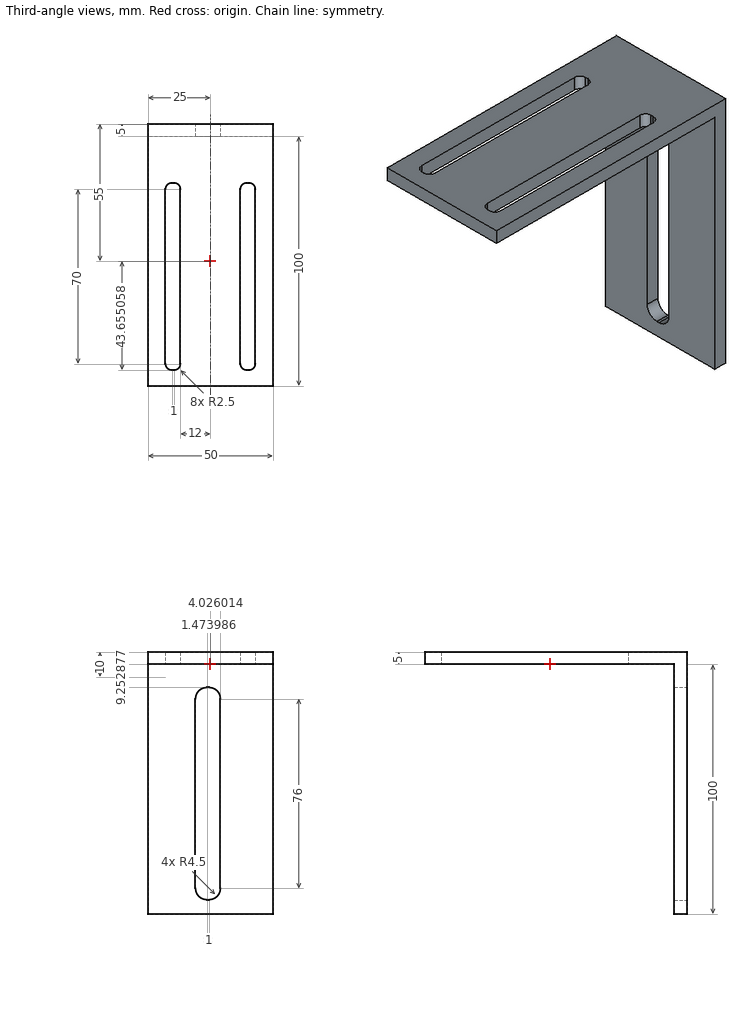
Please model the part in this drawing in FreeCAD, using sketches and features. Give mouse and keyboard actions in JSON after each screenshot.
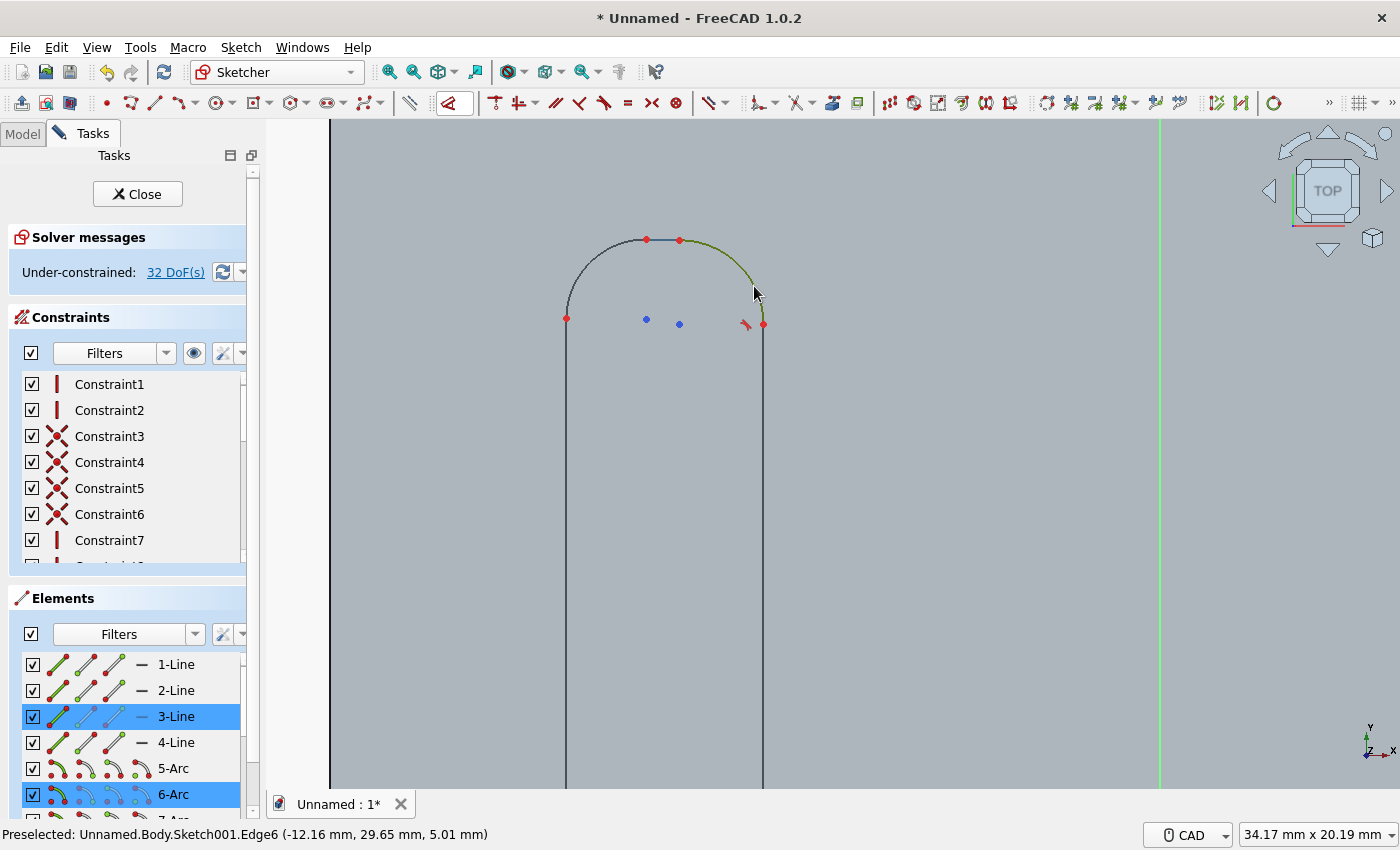
{"action": "key", "text": "t"}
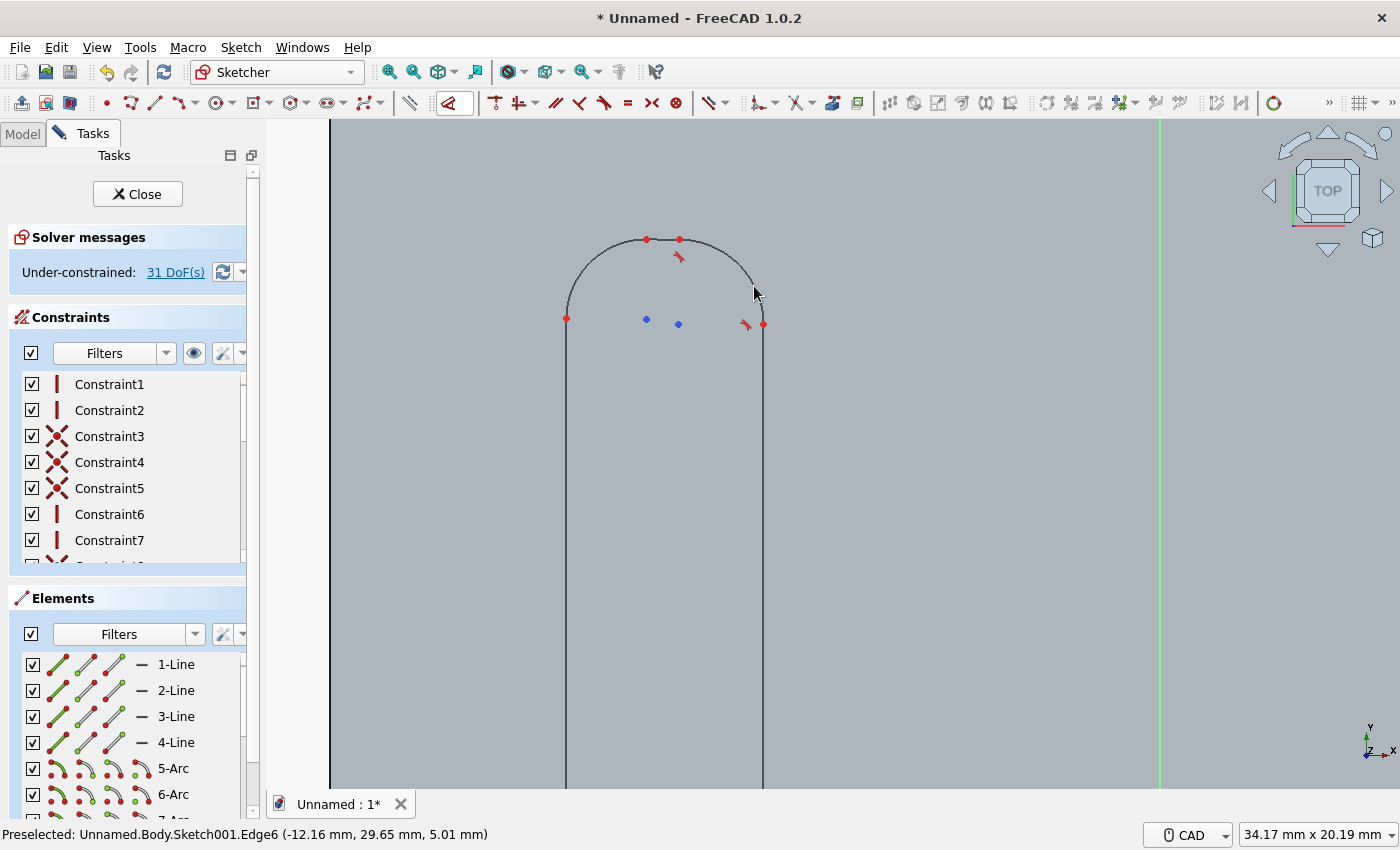
{"action": "scroll", "coordinate": [669, 240], "scroll_direction": "up", "scroll_amount": 2}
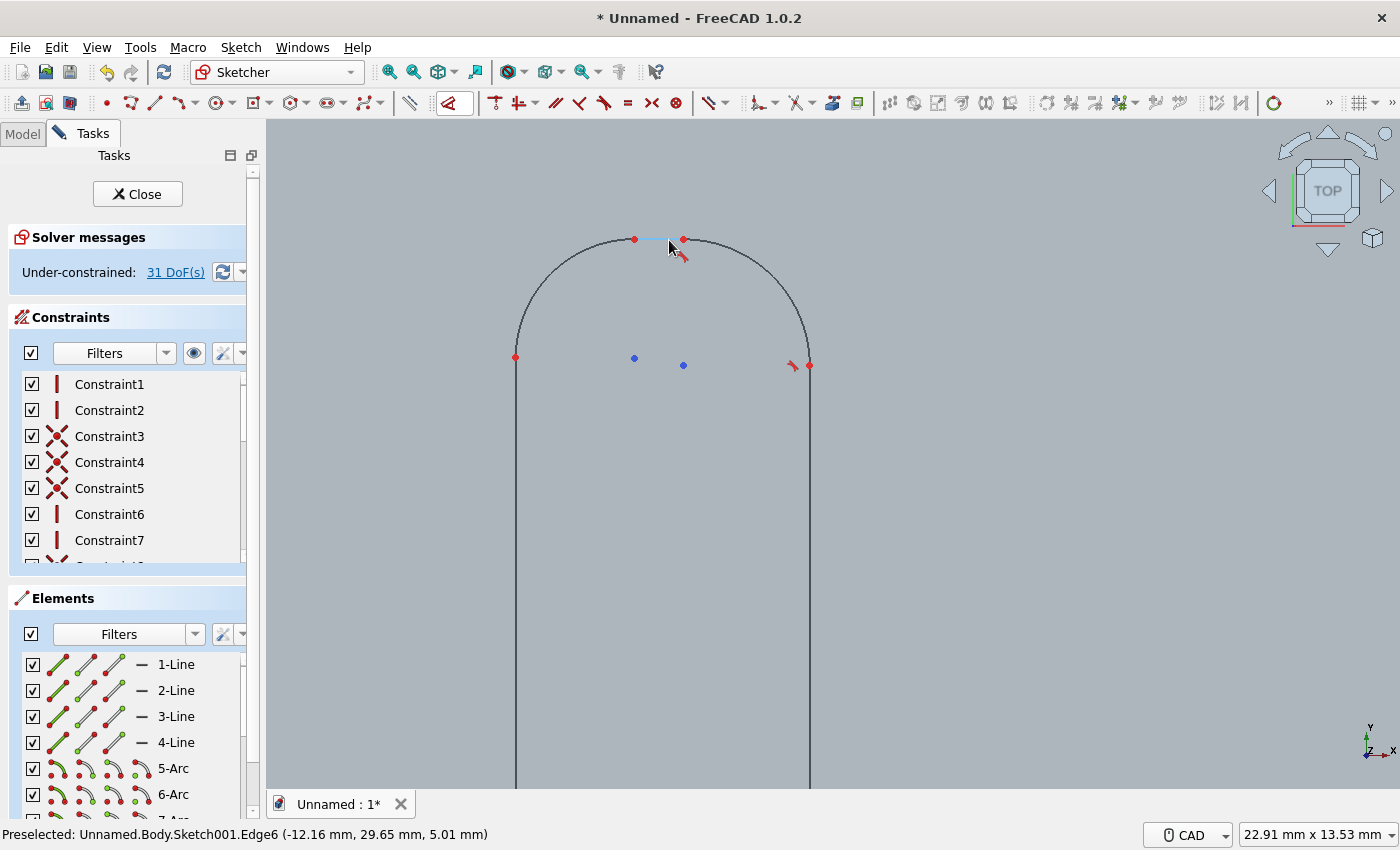
{"action": "left_click", "coordinate": [669, 239]}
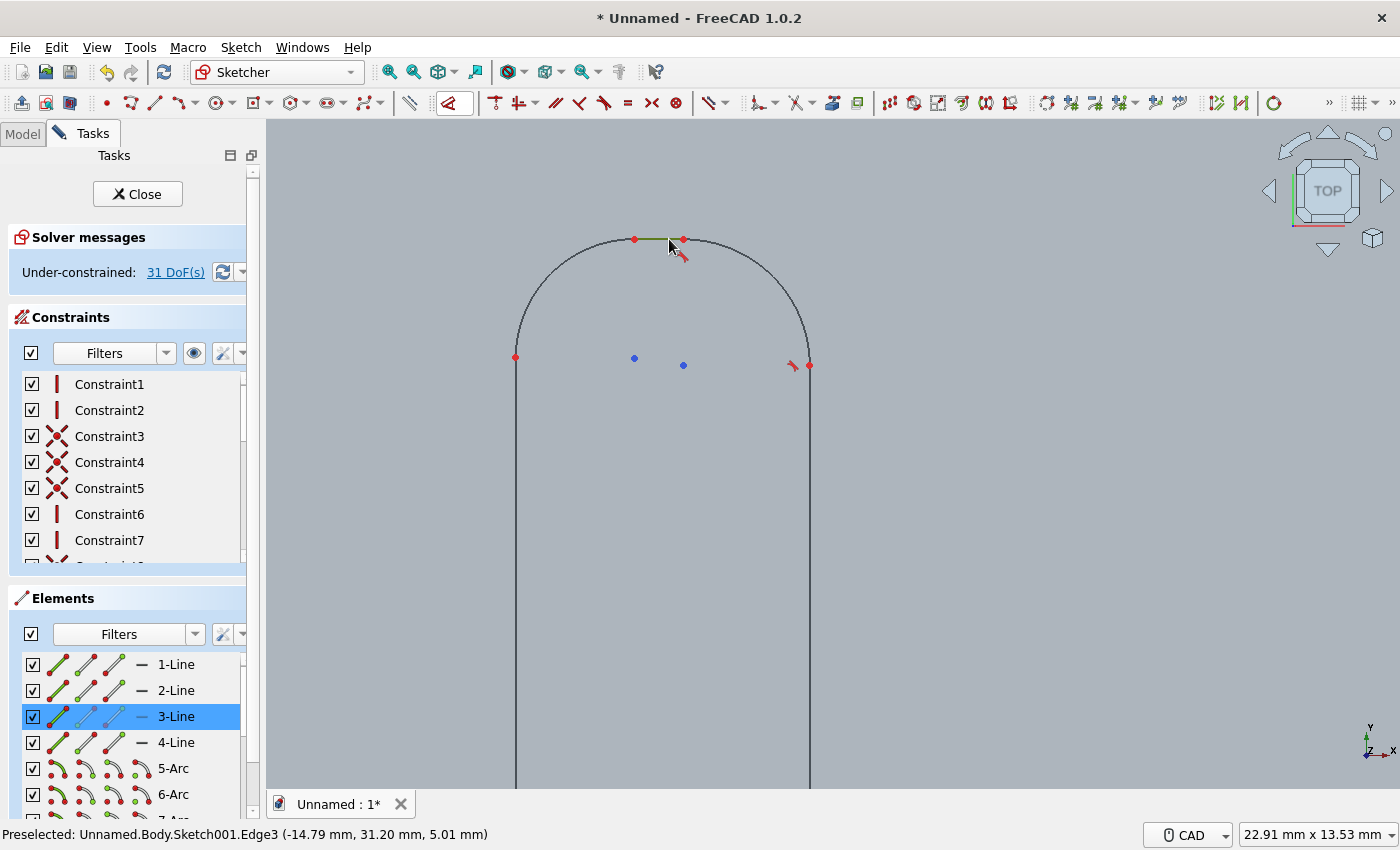
{"action": "scroll", "coordinate": [685, 250], "scroll_direction": "down", "scroll_amount": 11}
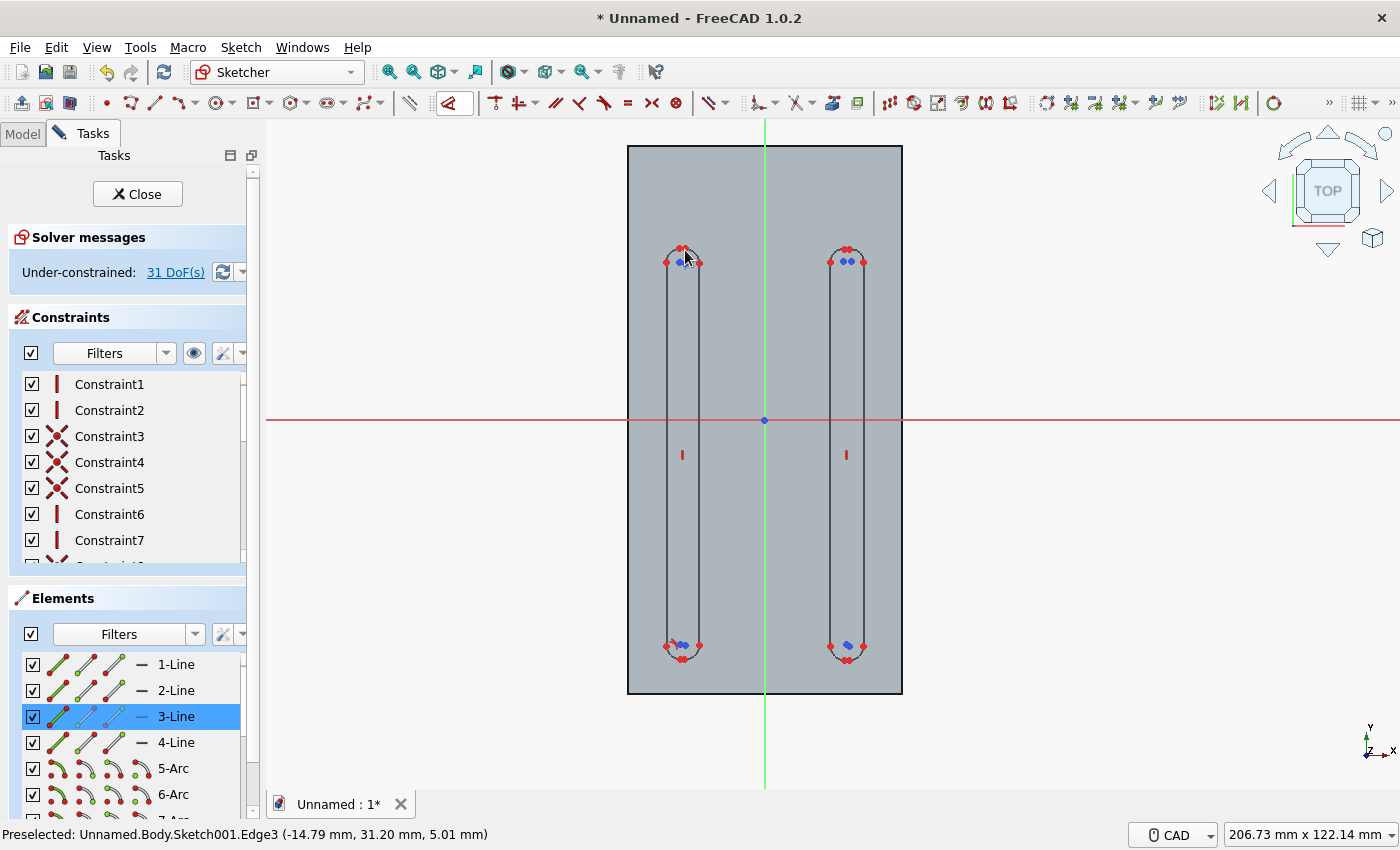
{"action": "scroll", "coordinate": [674, 250], "scroll_direction": "up", "scroll_amount": 5}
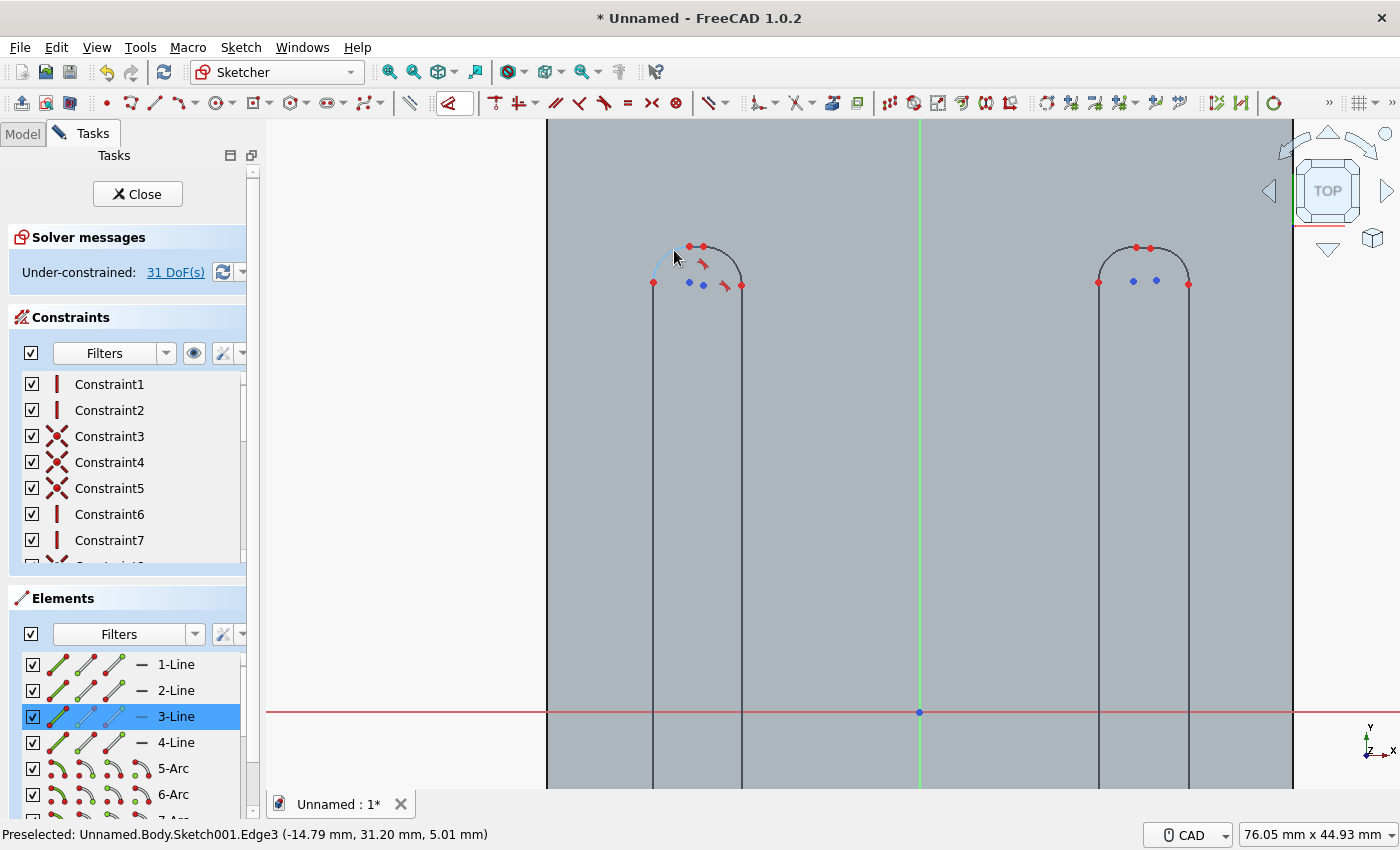
{"action": "left_click", "coordinate": [673, 251]}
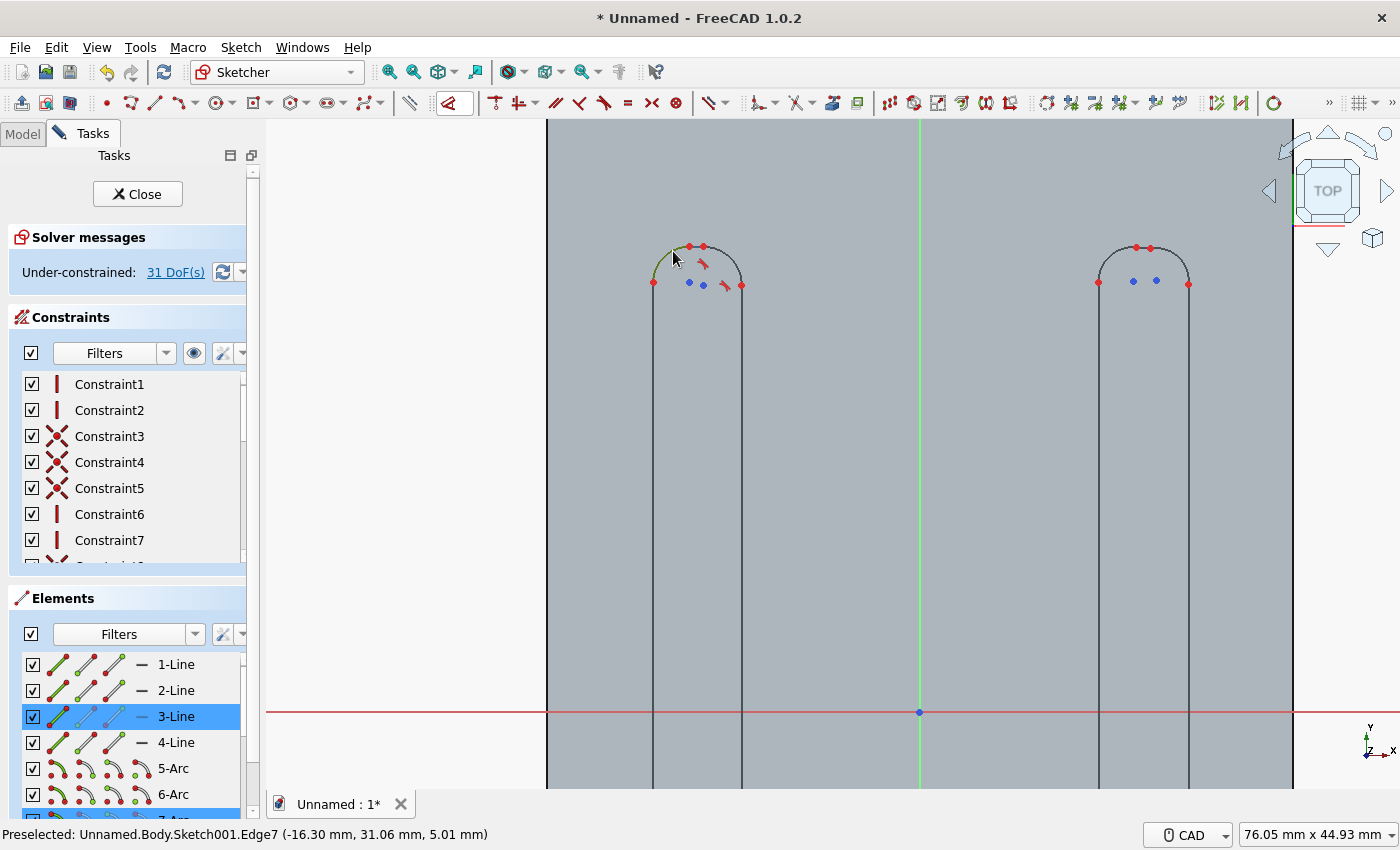
{"action": "key", "text": "t"}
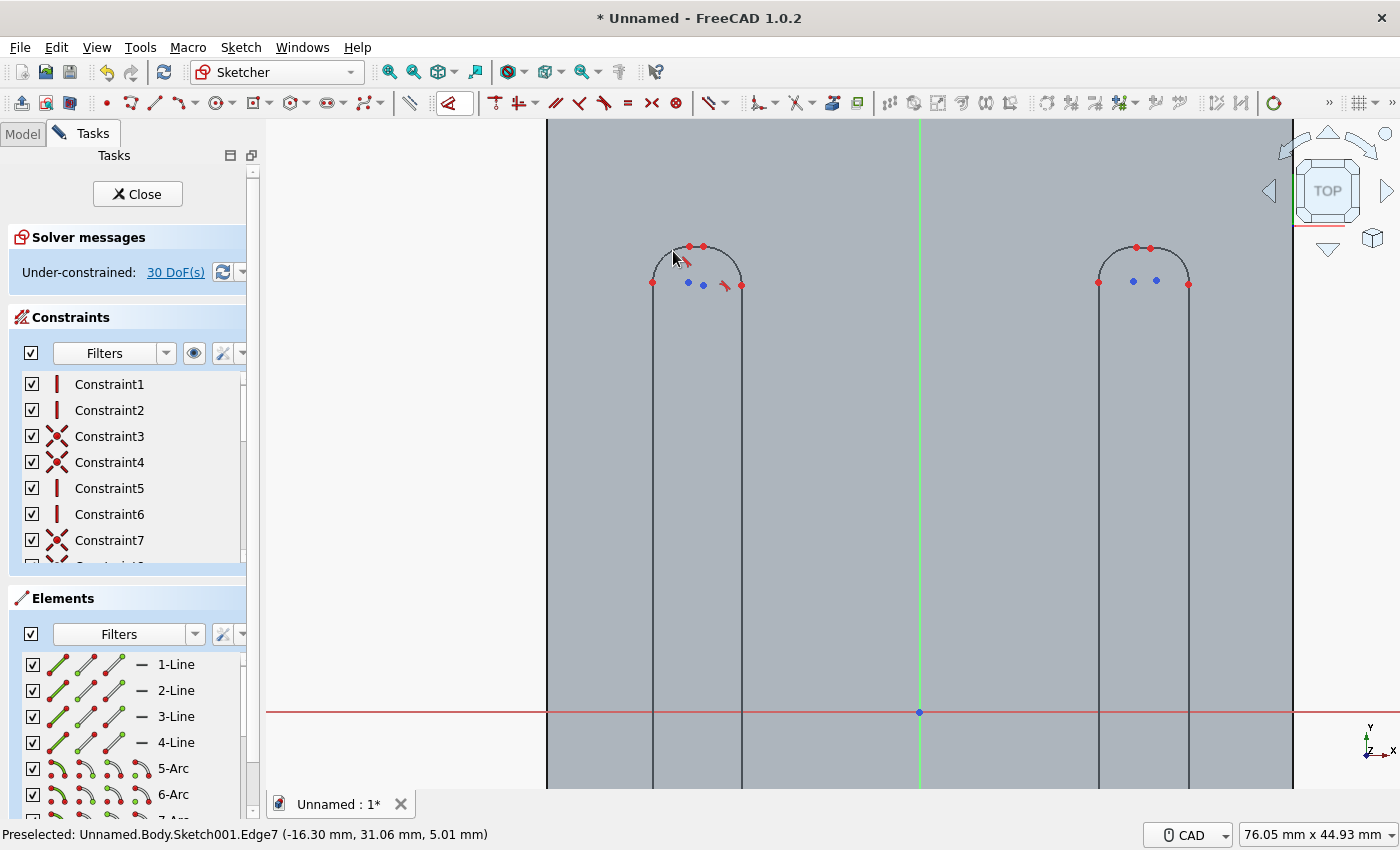
{"action": "left_click", "coordinate": [653, 596]}